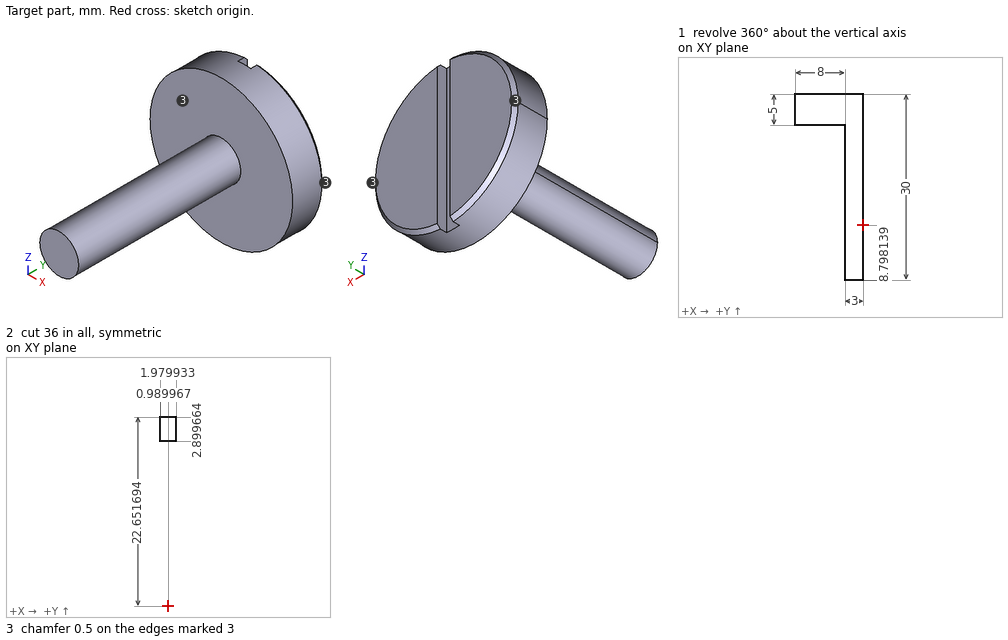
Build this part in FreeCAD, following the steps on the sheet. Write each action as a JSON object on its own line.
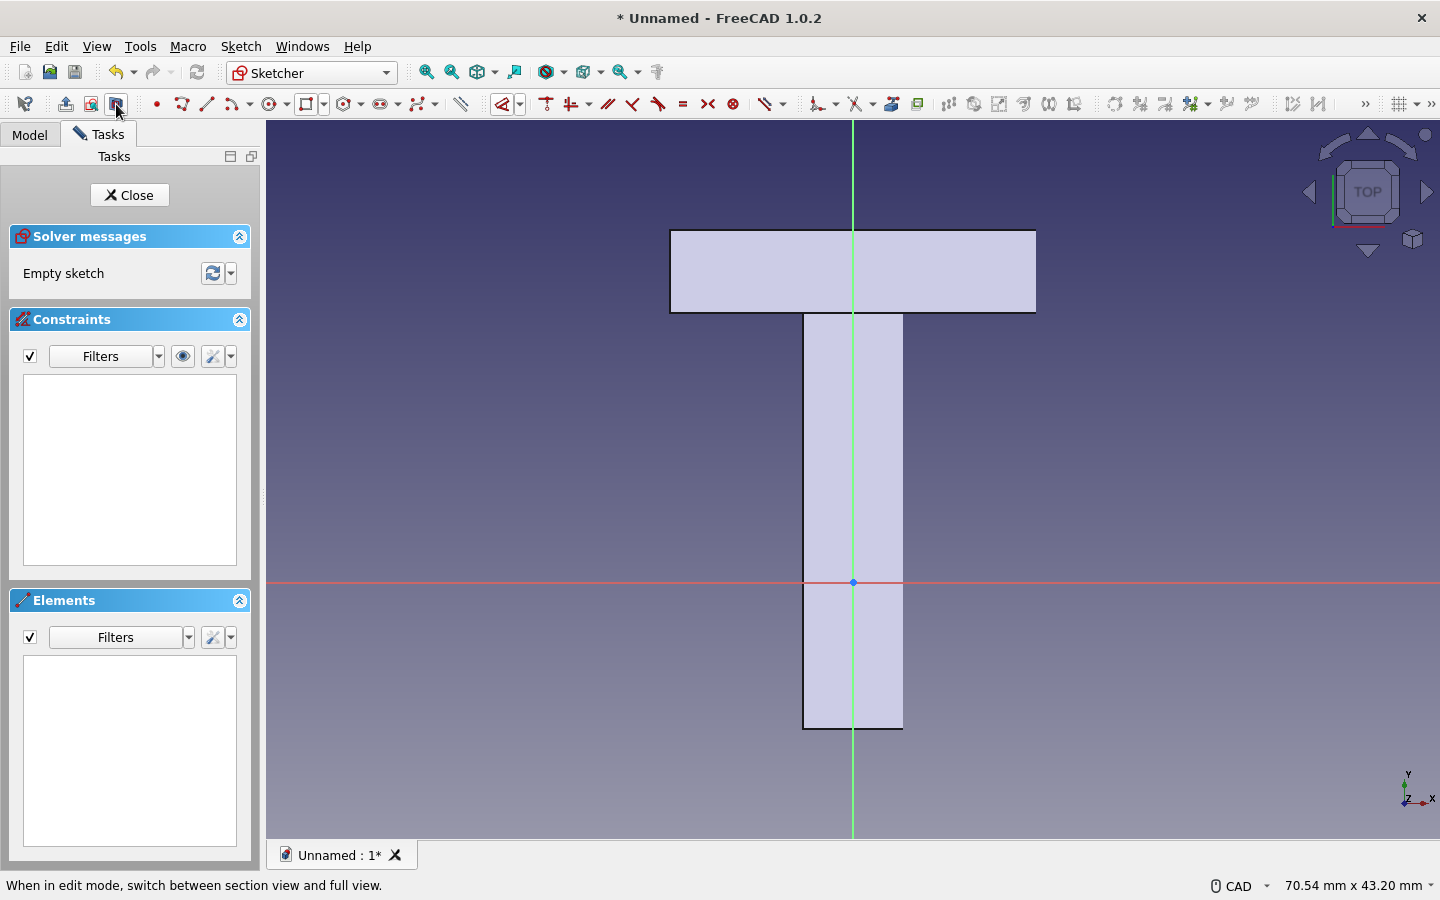
{"action": "scroll", "coordinate": [862, 199], "scroll_direction": "up", "scroll_amount": 11}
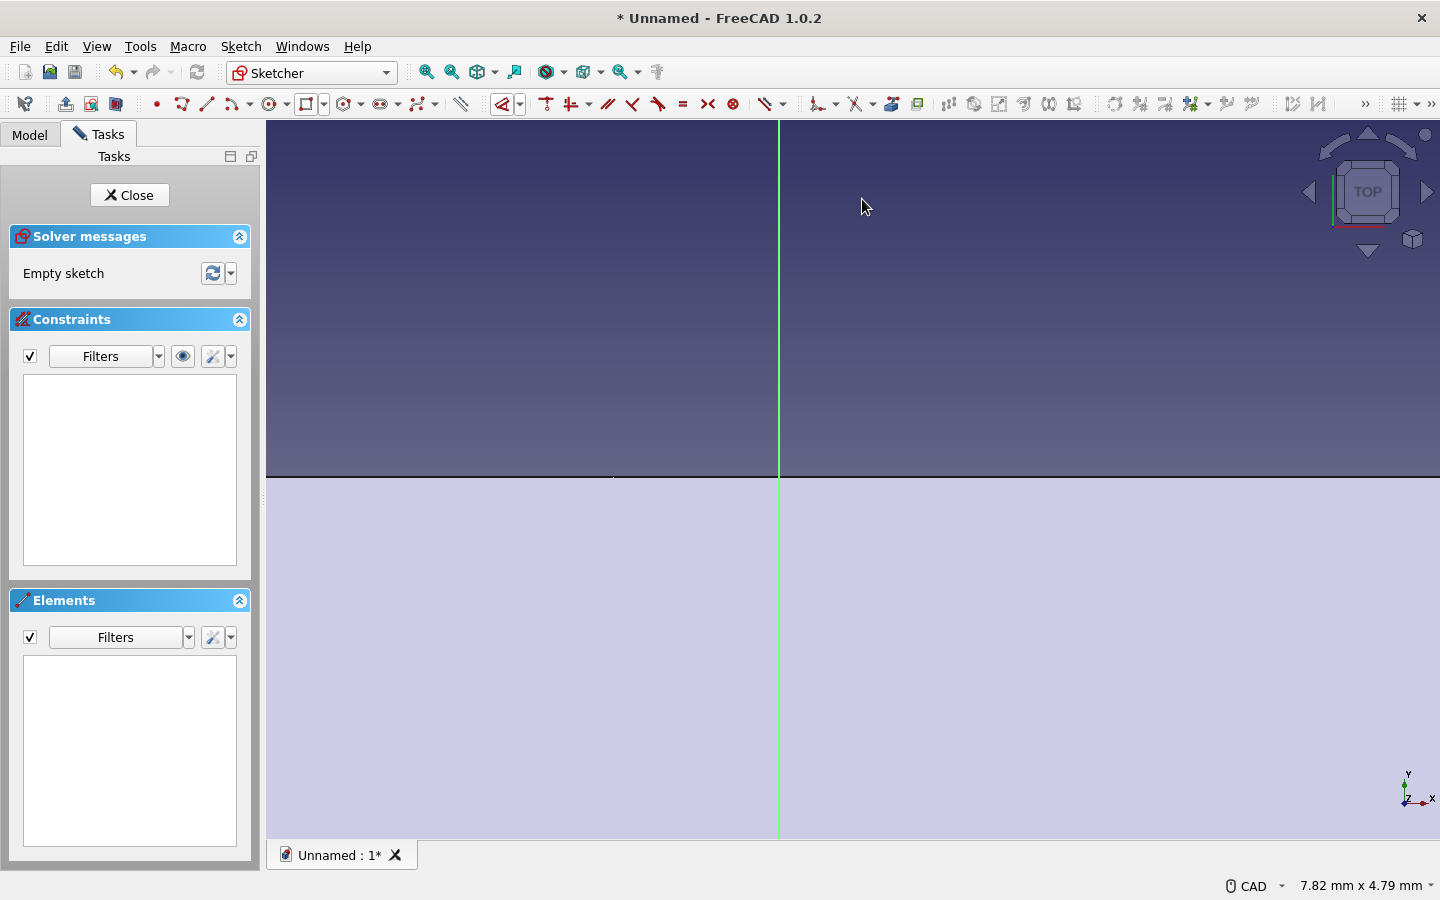
{"action": "left_click", "coordinate": [306, 104]}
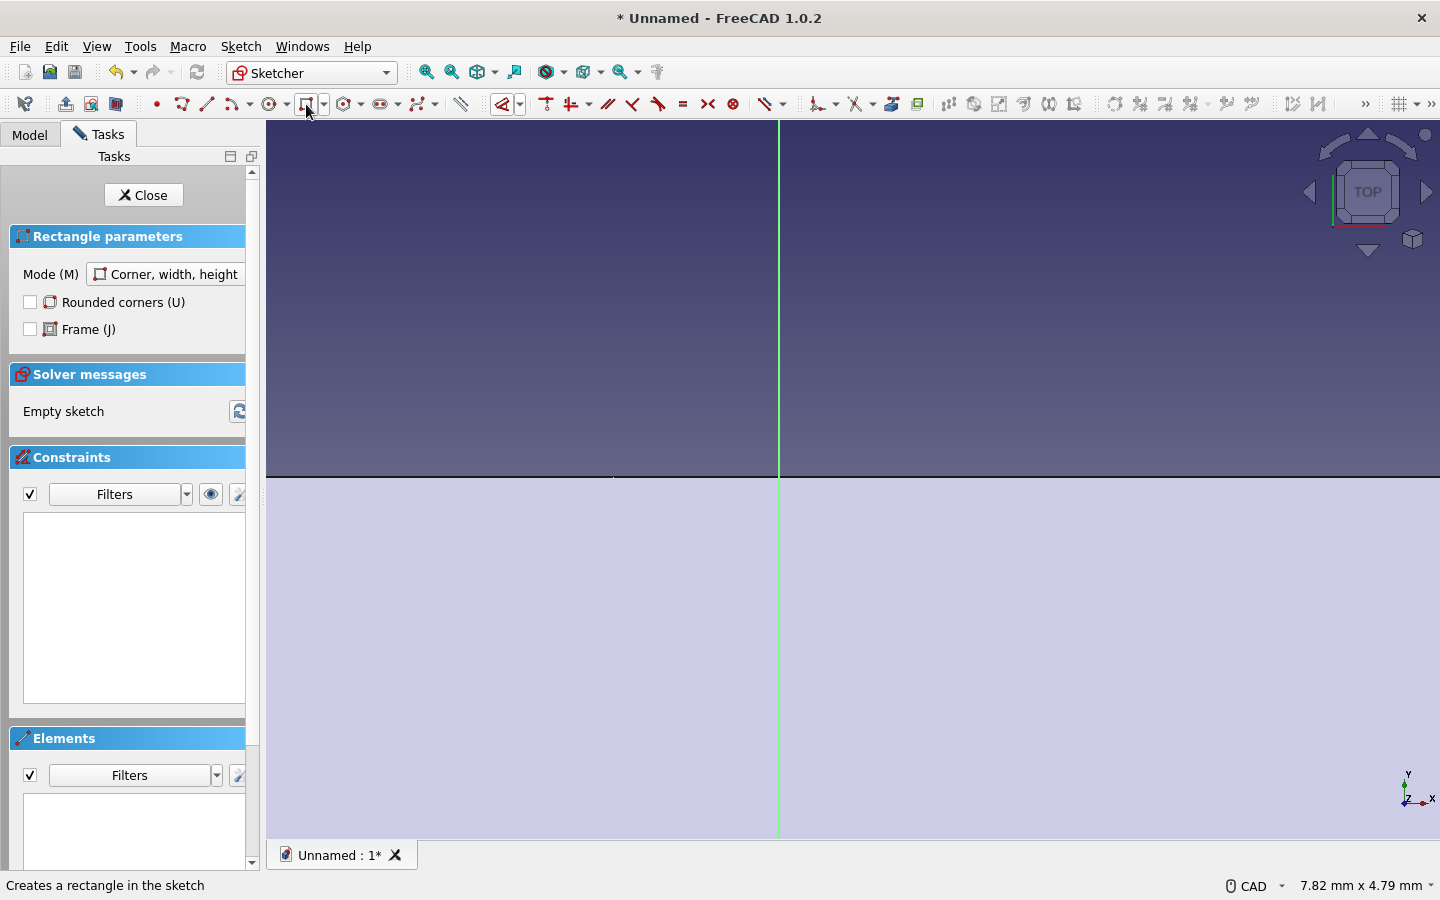
{"action": "left_click", "coordinate": [630, 259]}
{"action": "mouse_move", "coordinate": [927, 694]}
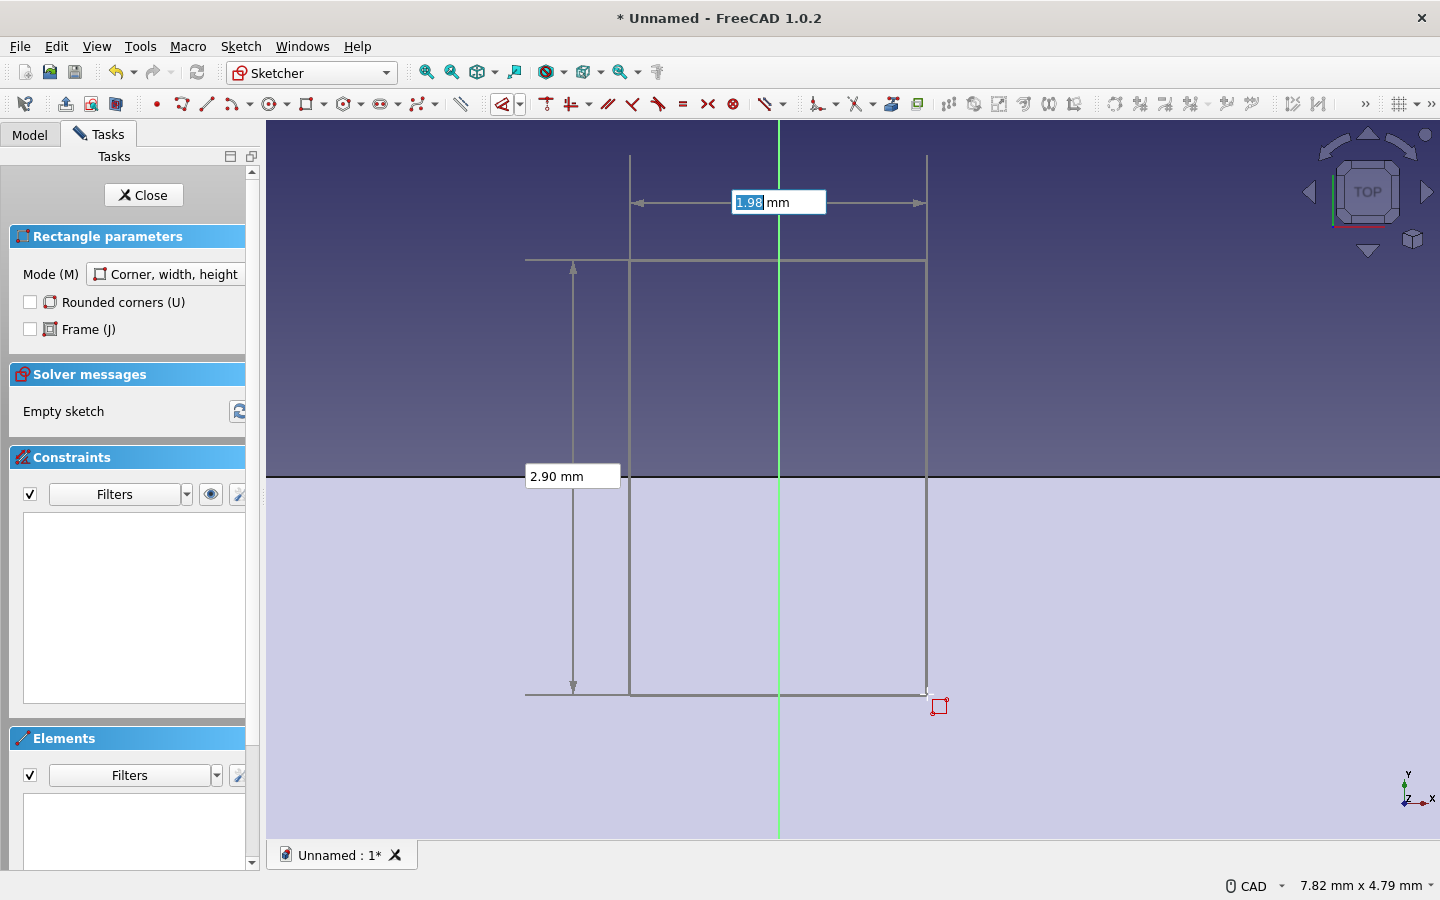
{"action": "type", "text": "1.979933"}
{"action": "key", "text": "Tab"}
{"action": "type", "text": "2.899664"}
{"action": "key", "text": "Return"}
{"action": "key", "text": "Escape"}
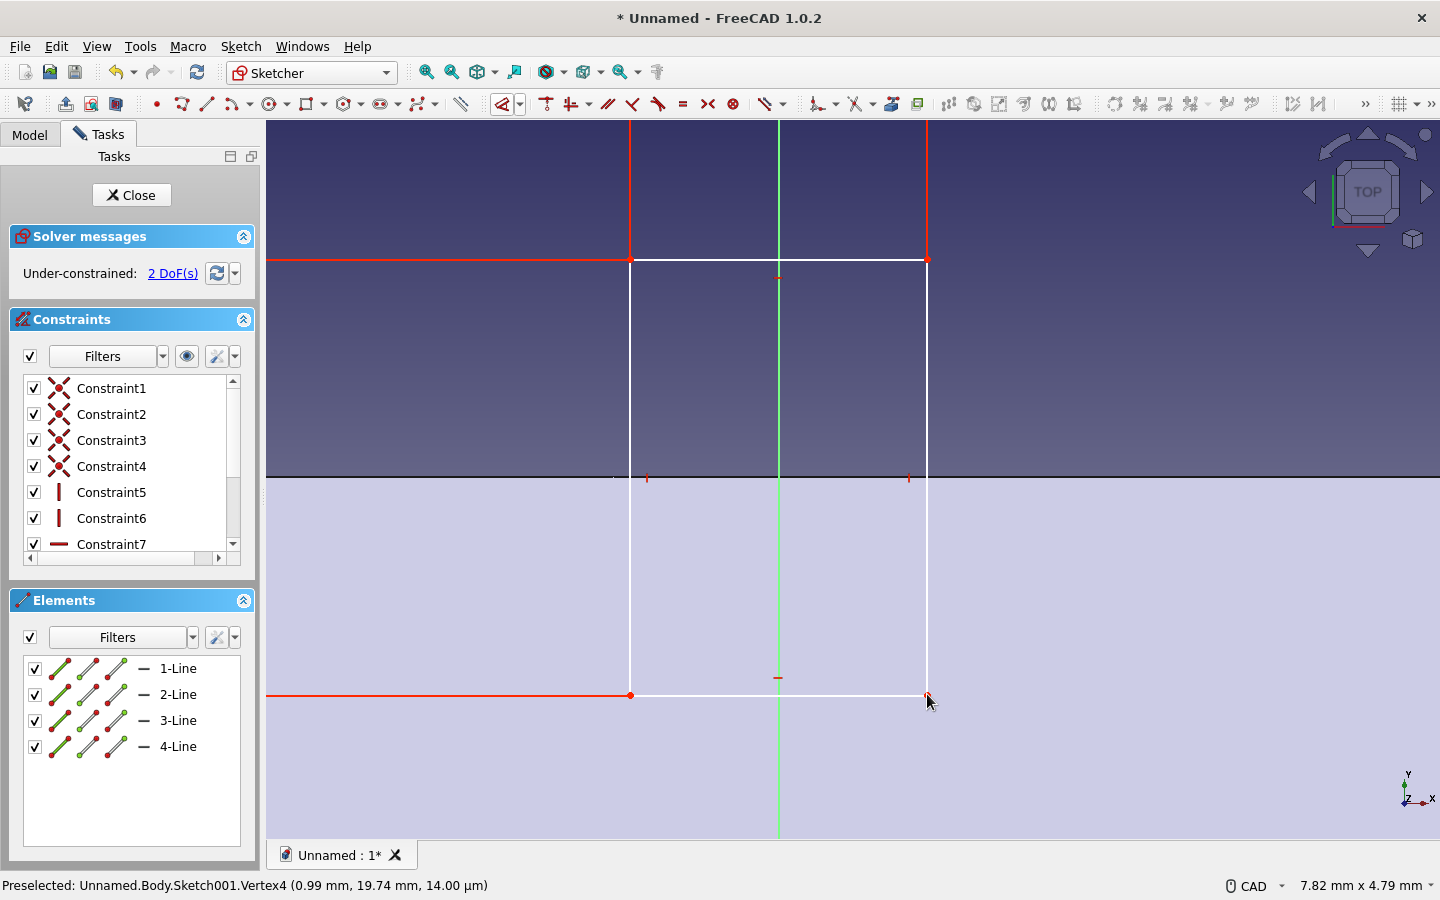
{"action": "left_click", "coordinate": [630, 260]}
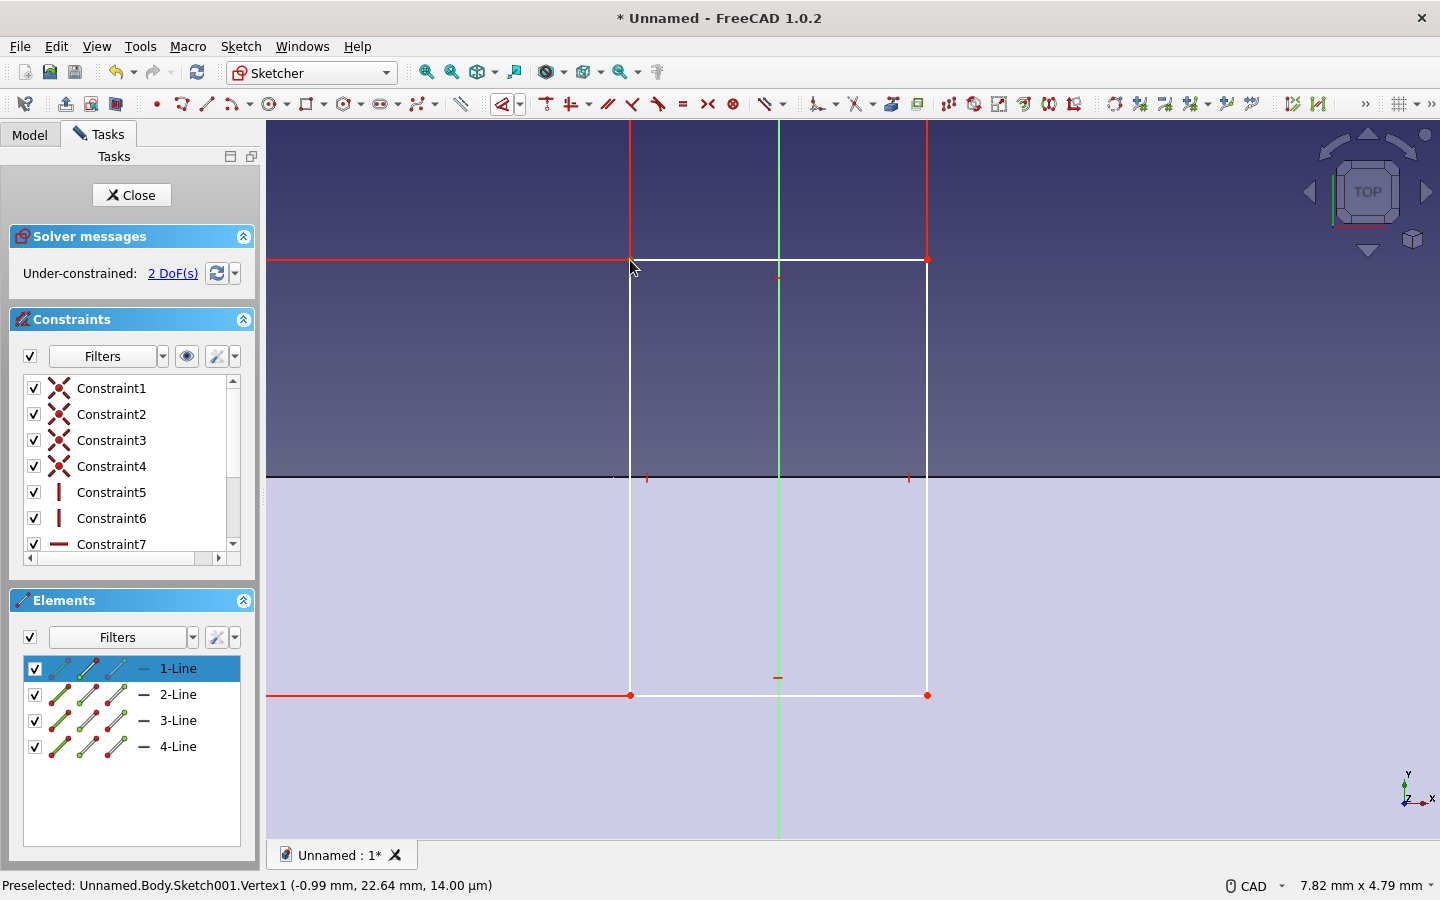
{"action": "left_click", "coordinate": [520, 104]}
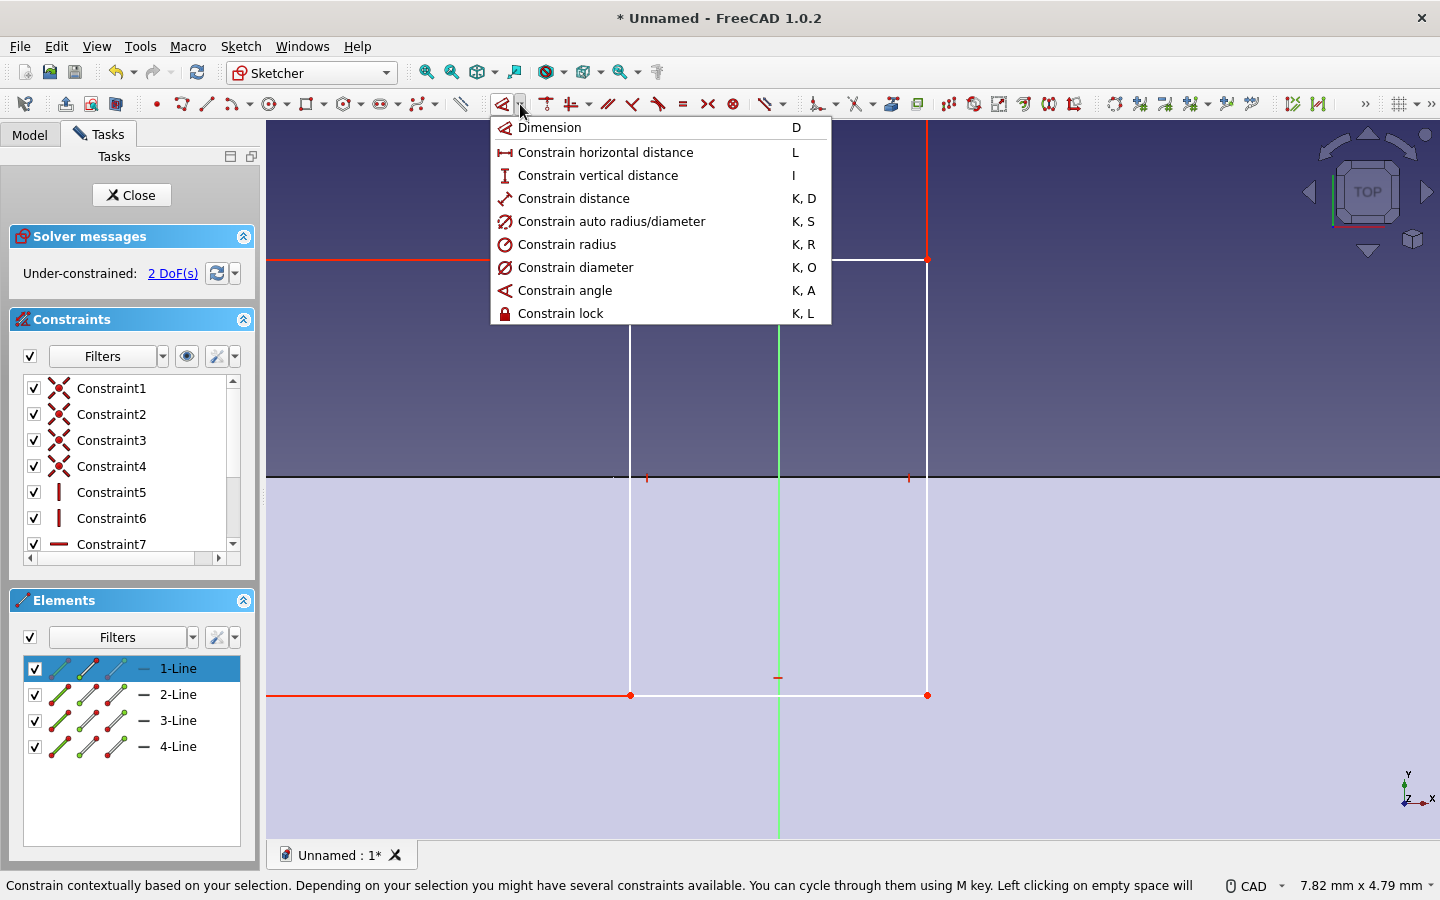
{"action": "left_click", "coordinate": [661, 152]}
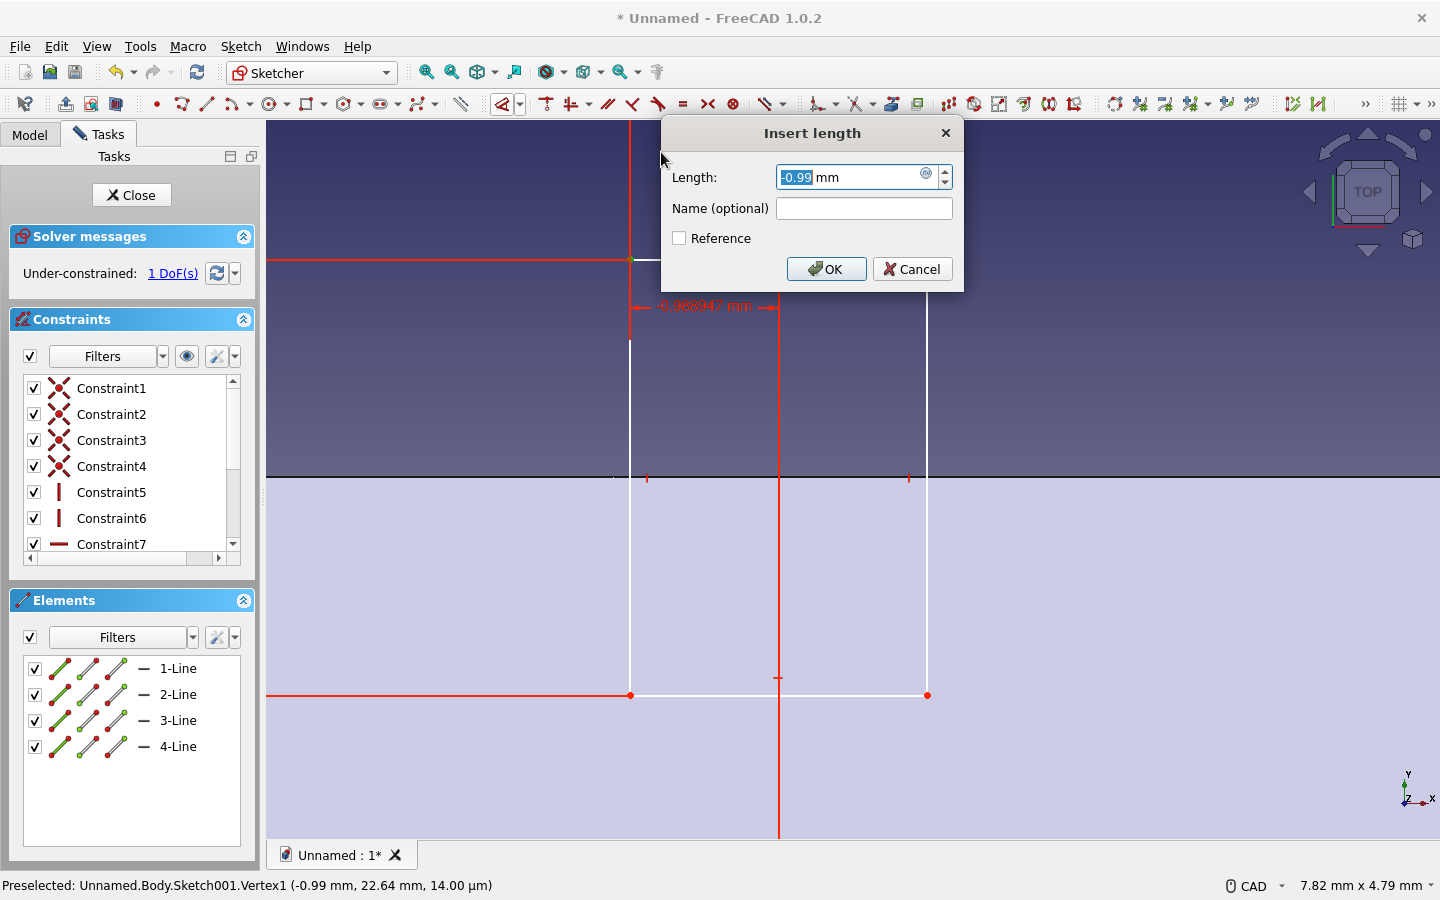
{"action": "type", "text": "-0.989967"}
{"action": "key", "text": "Return"}